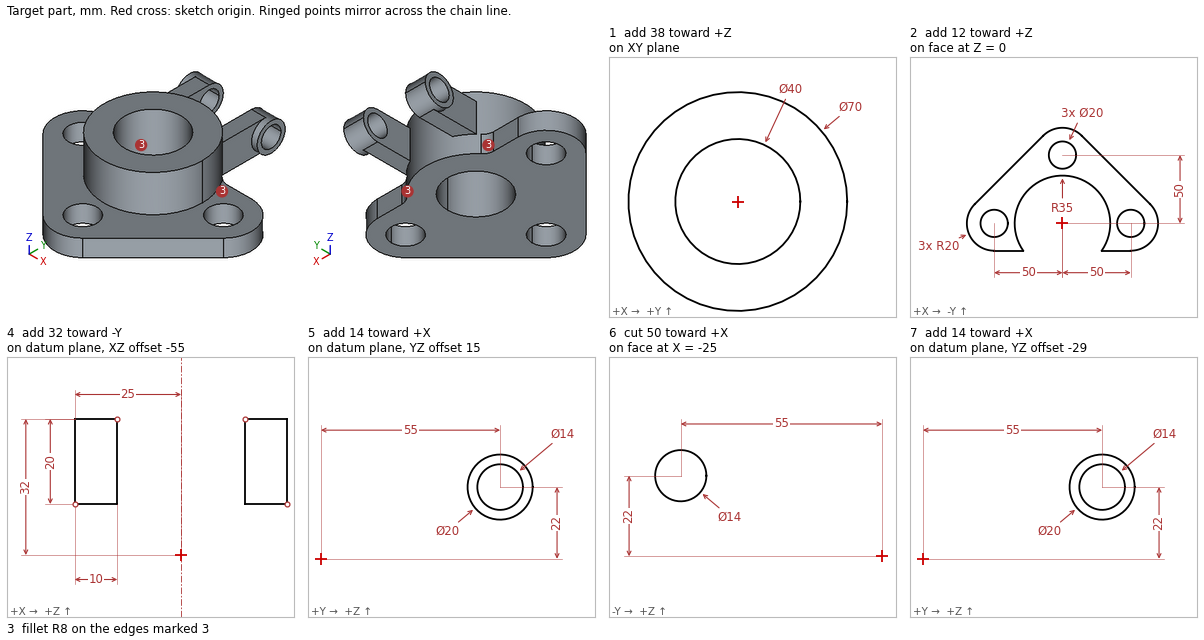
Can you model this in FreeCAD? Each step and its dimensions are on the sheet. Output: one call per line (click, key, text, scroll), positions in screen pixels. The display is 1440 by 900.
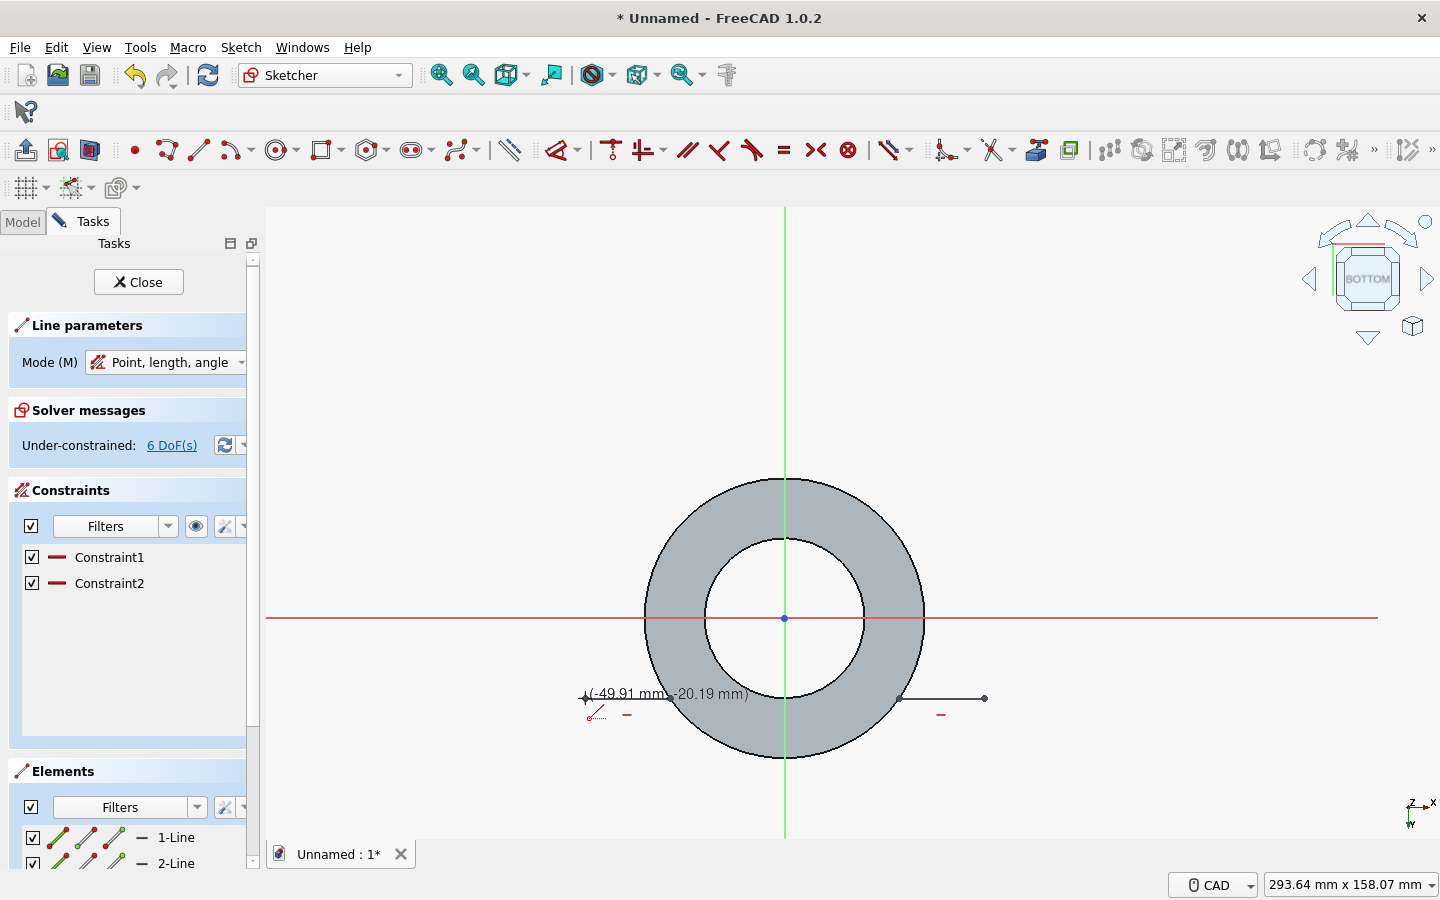
click(528, 562)
click(728, 362)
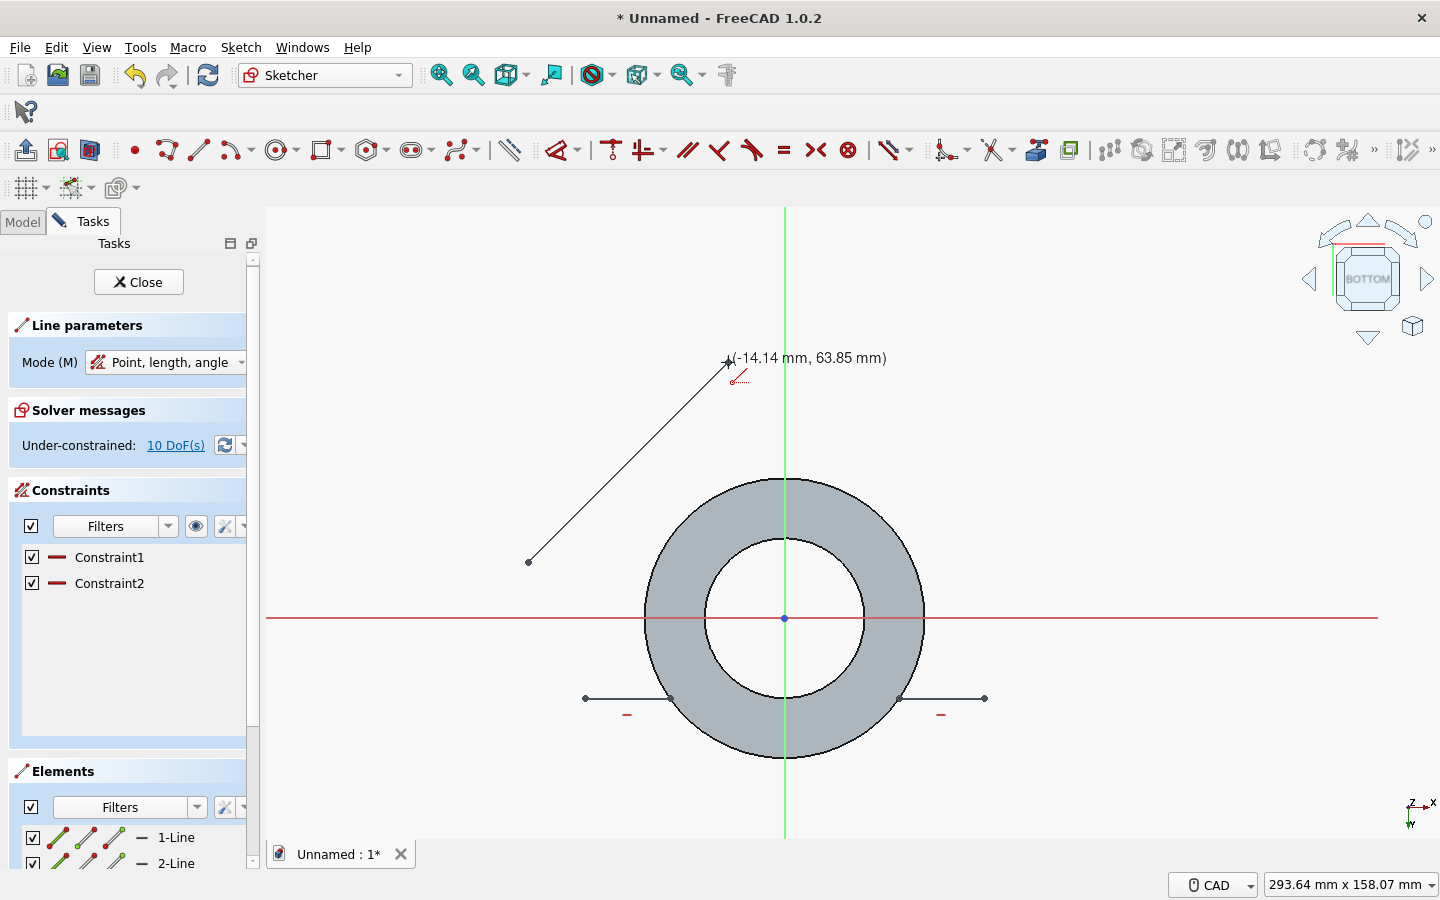
click(841, 362)
click(1041, 562)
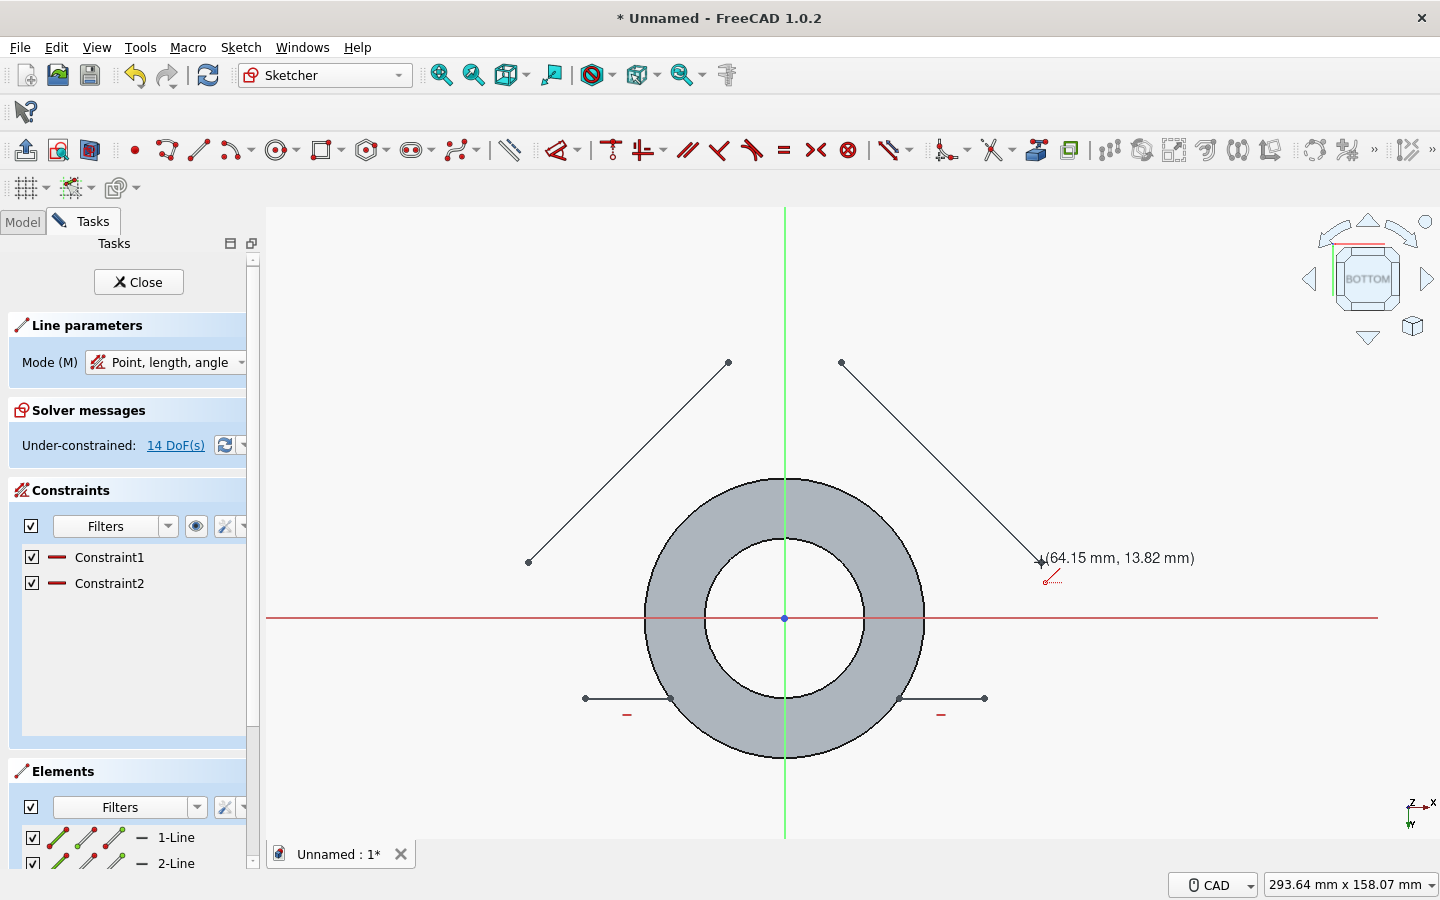
key(g)
key(3)
key(a)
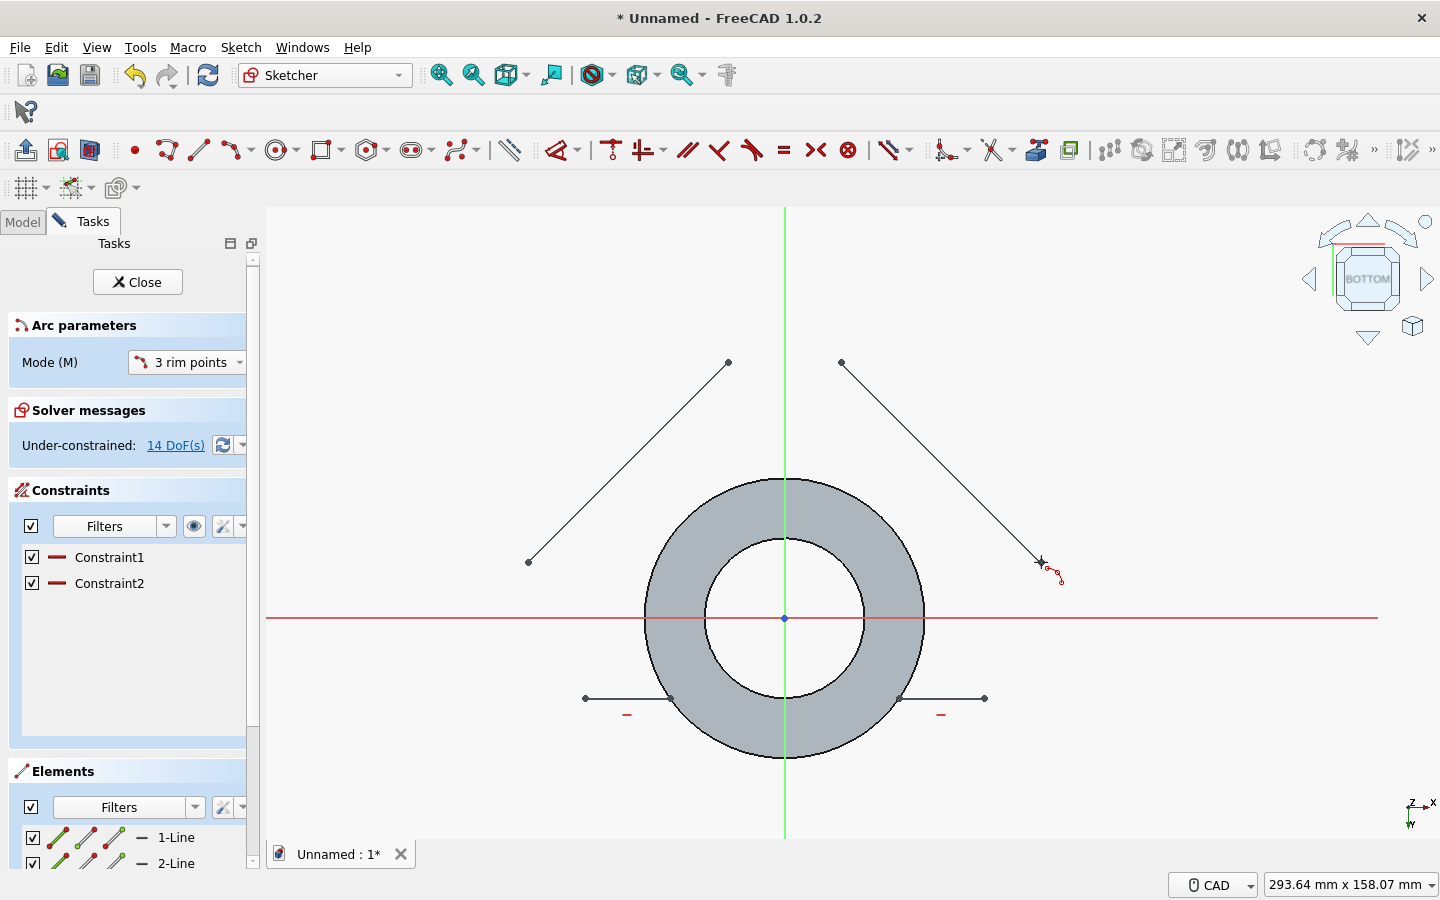
click(899, 699)
click(670, 699)
click(844, 491)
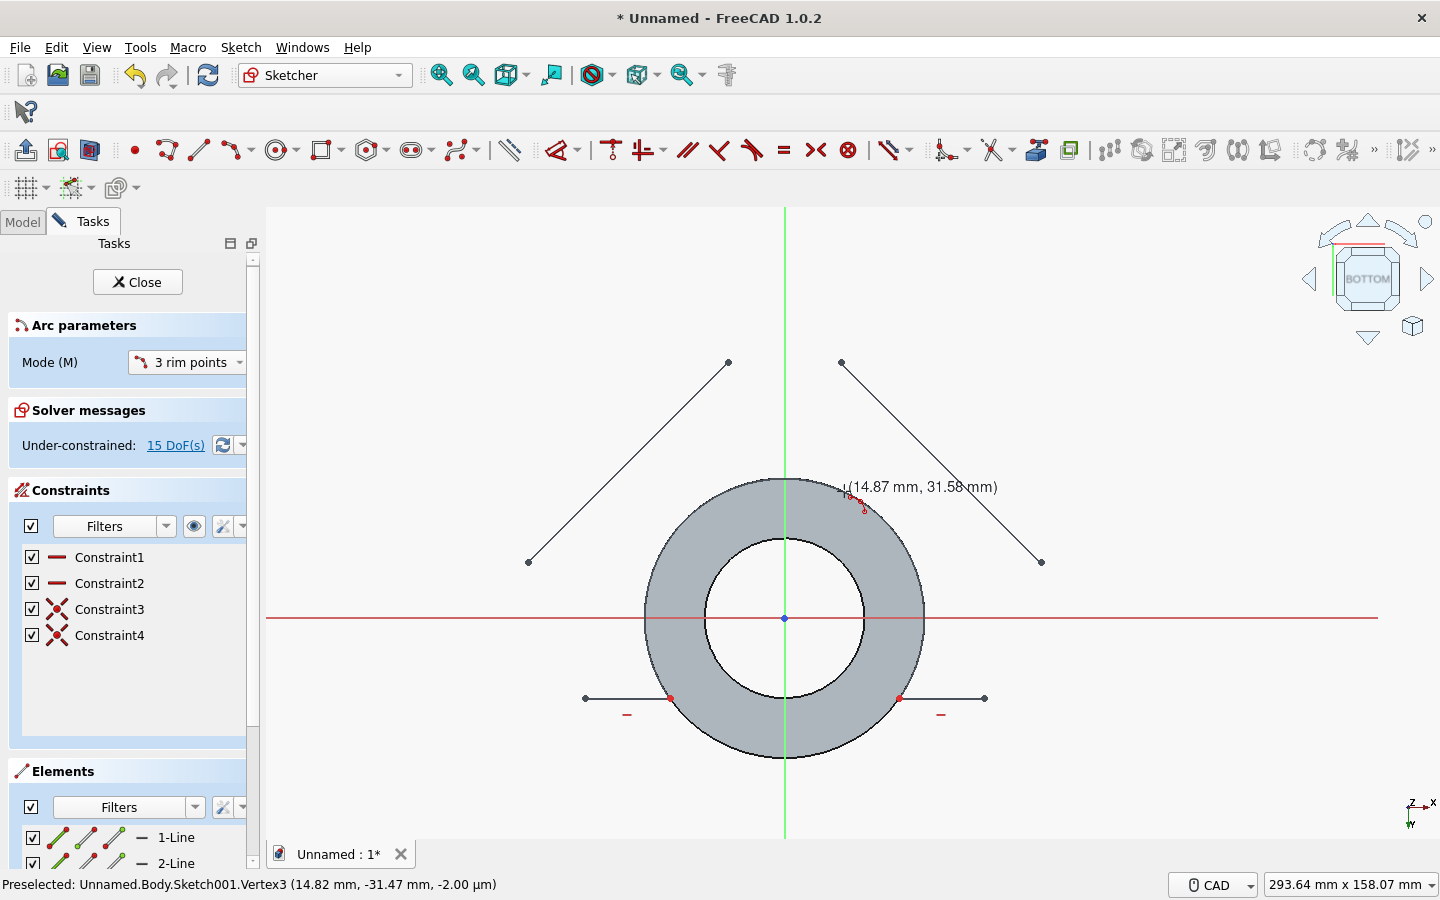
click(585, 699)
click(528, 563)
click(511, 649)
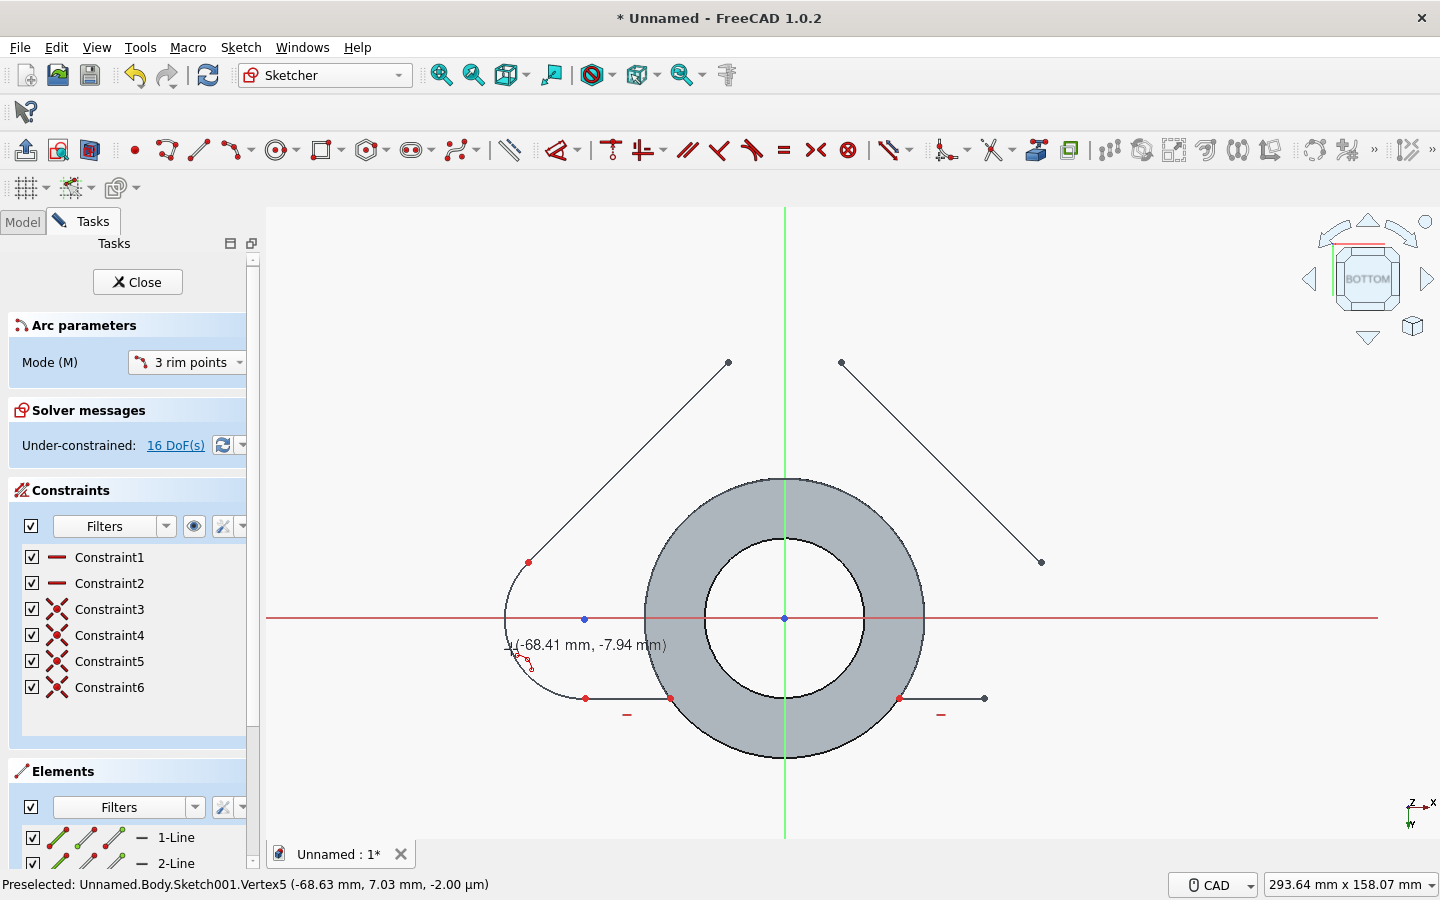
click(728, 363)
click(841, 363)
click(809, 342)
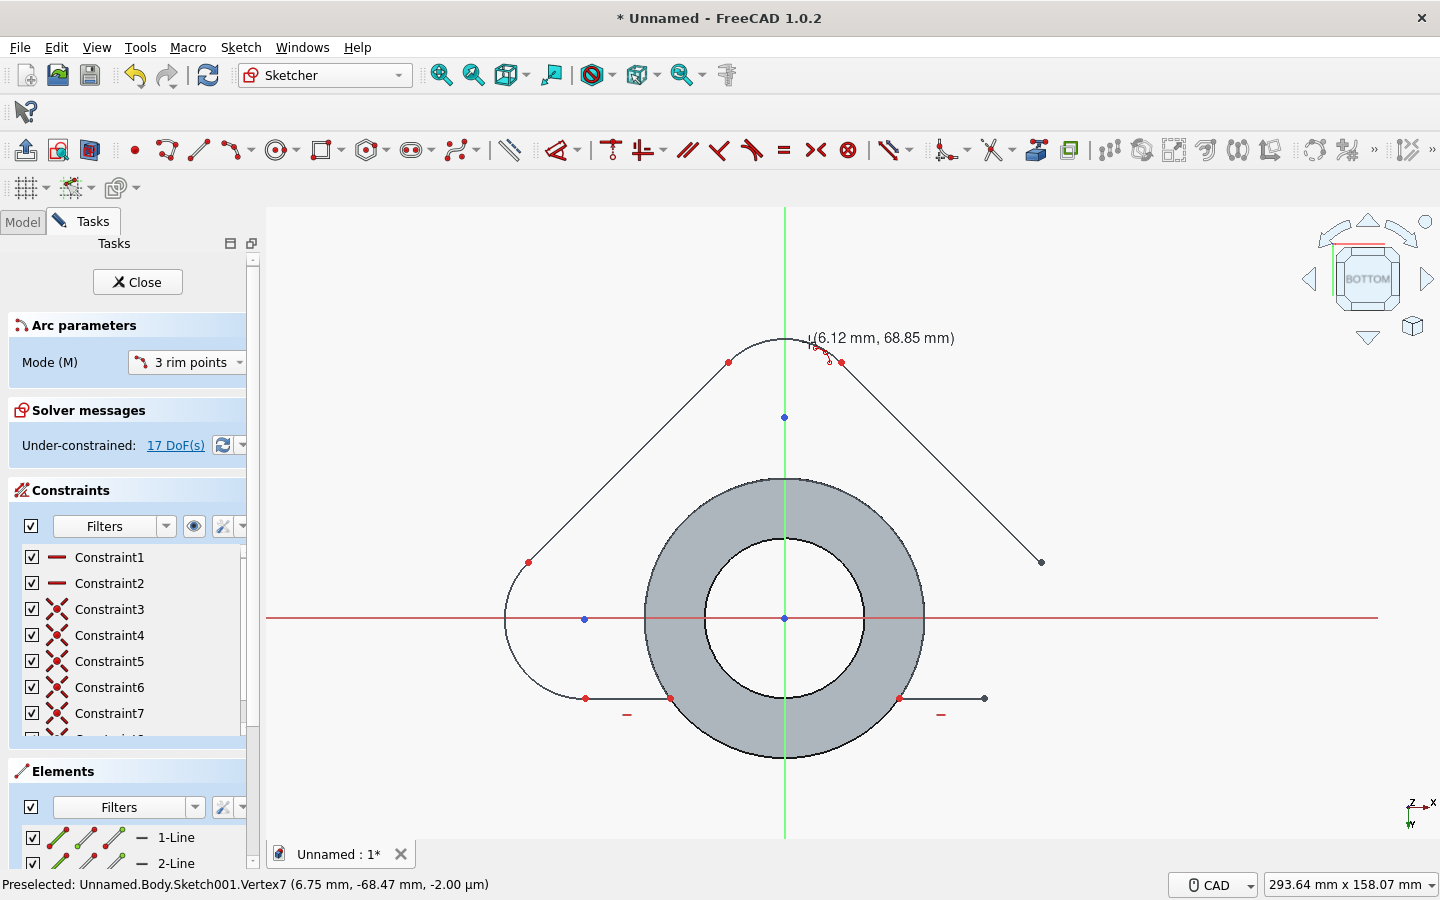
click(1041, 563)
click(984, 699)
click(1058, 649)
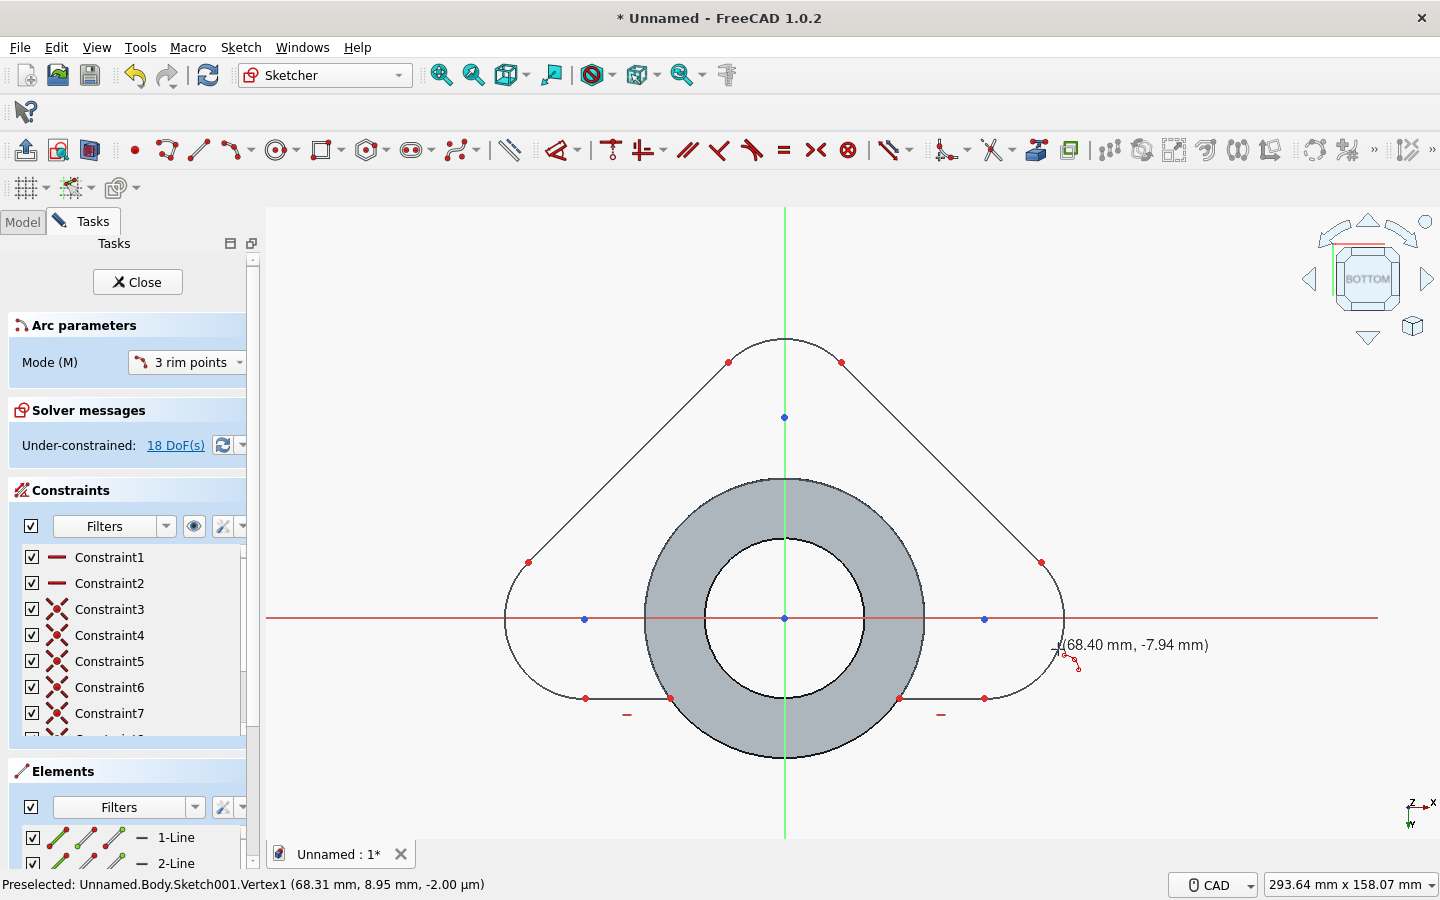
key(g)
key(c)